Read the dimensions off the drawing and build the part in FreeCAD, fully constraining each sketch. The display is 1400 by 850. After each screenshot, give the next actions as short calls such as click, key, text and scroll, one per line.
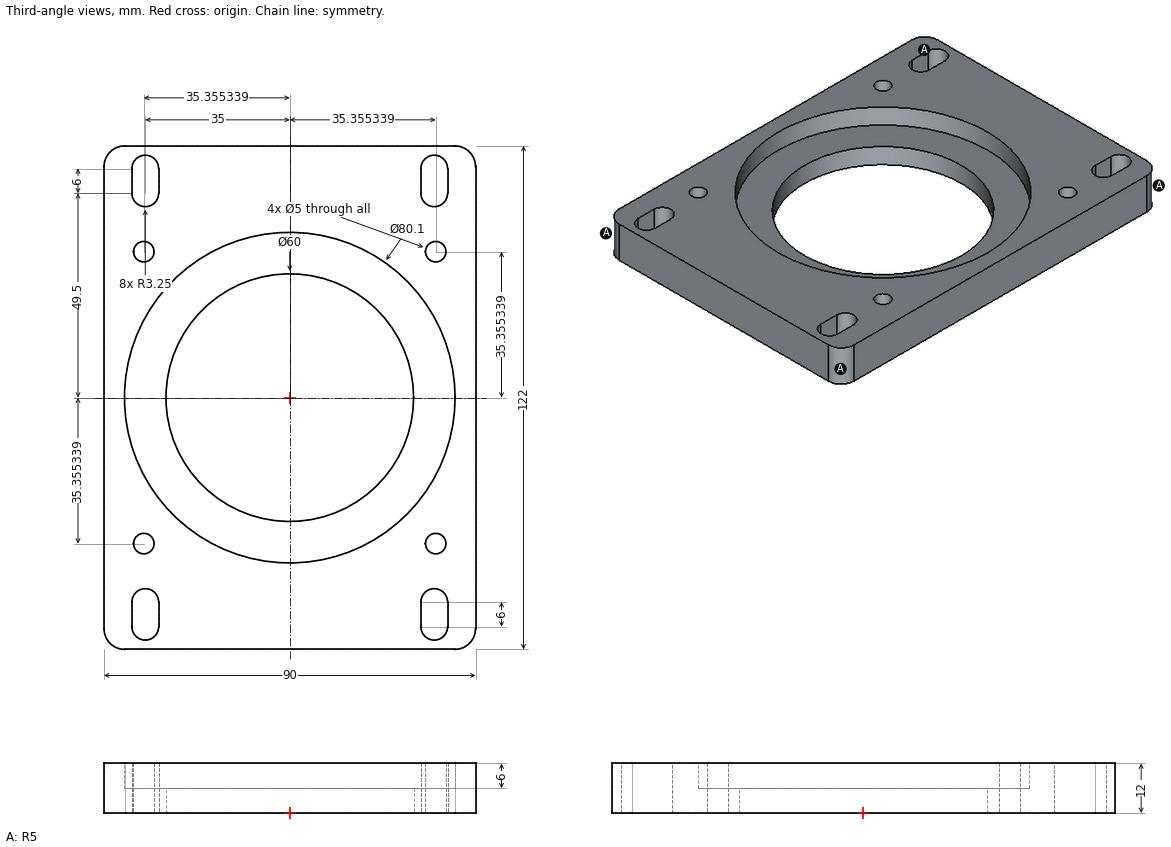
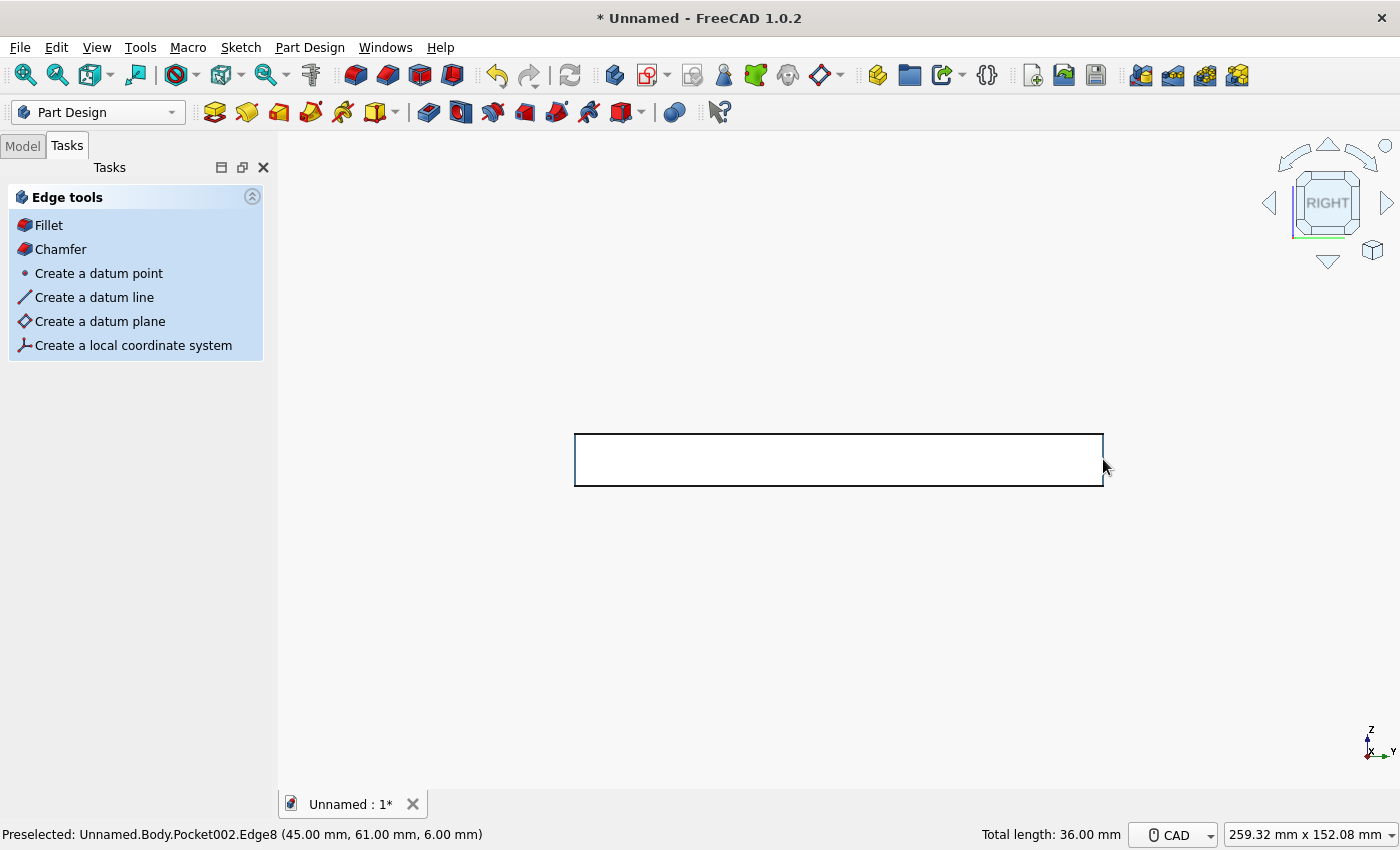
key(5)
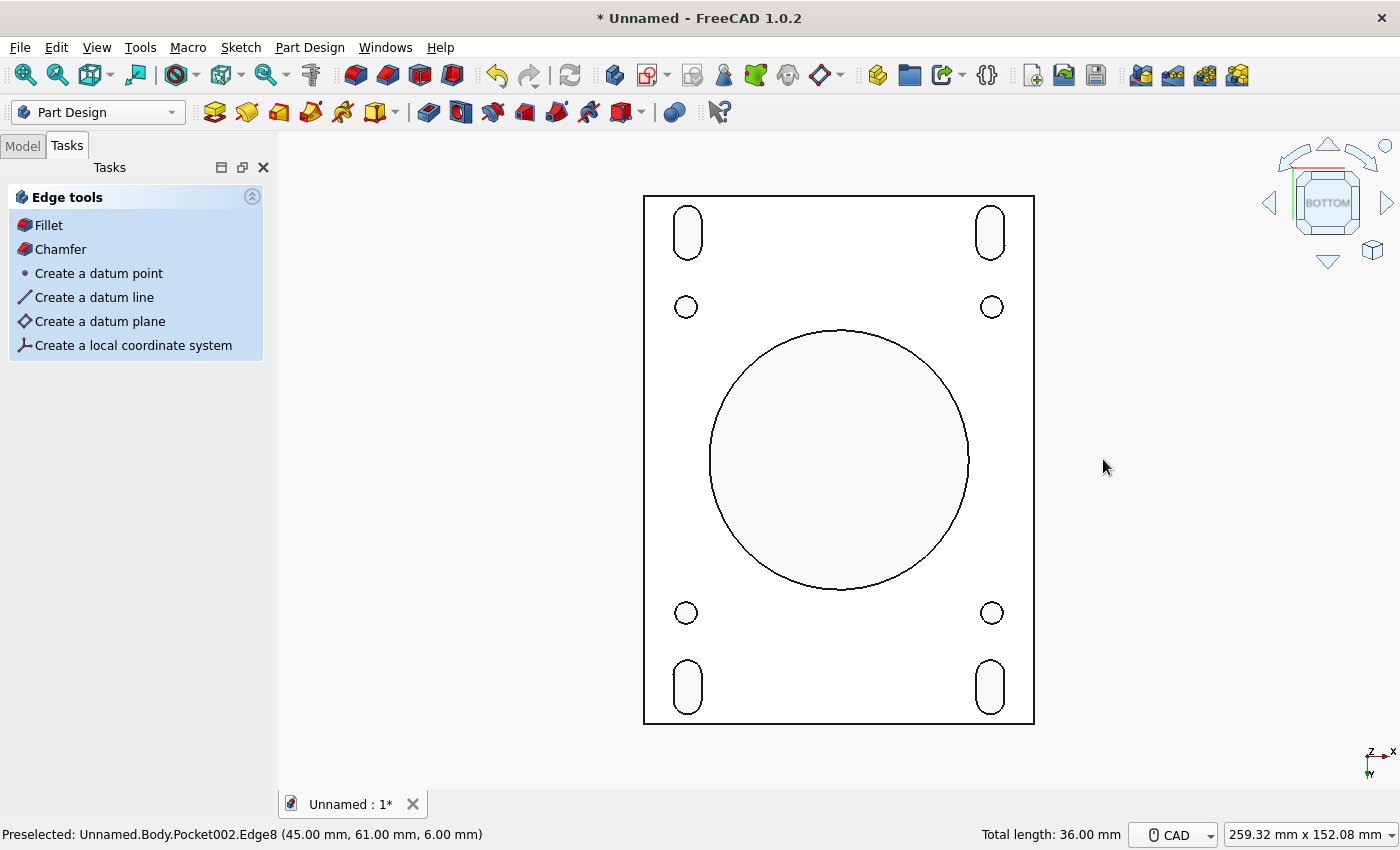
key(4)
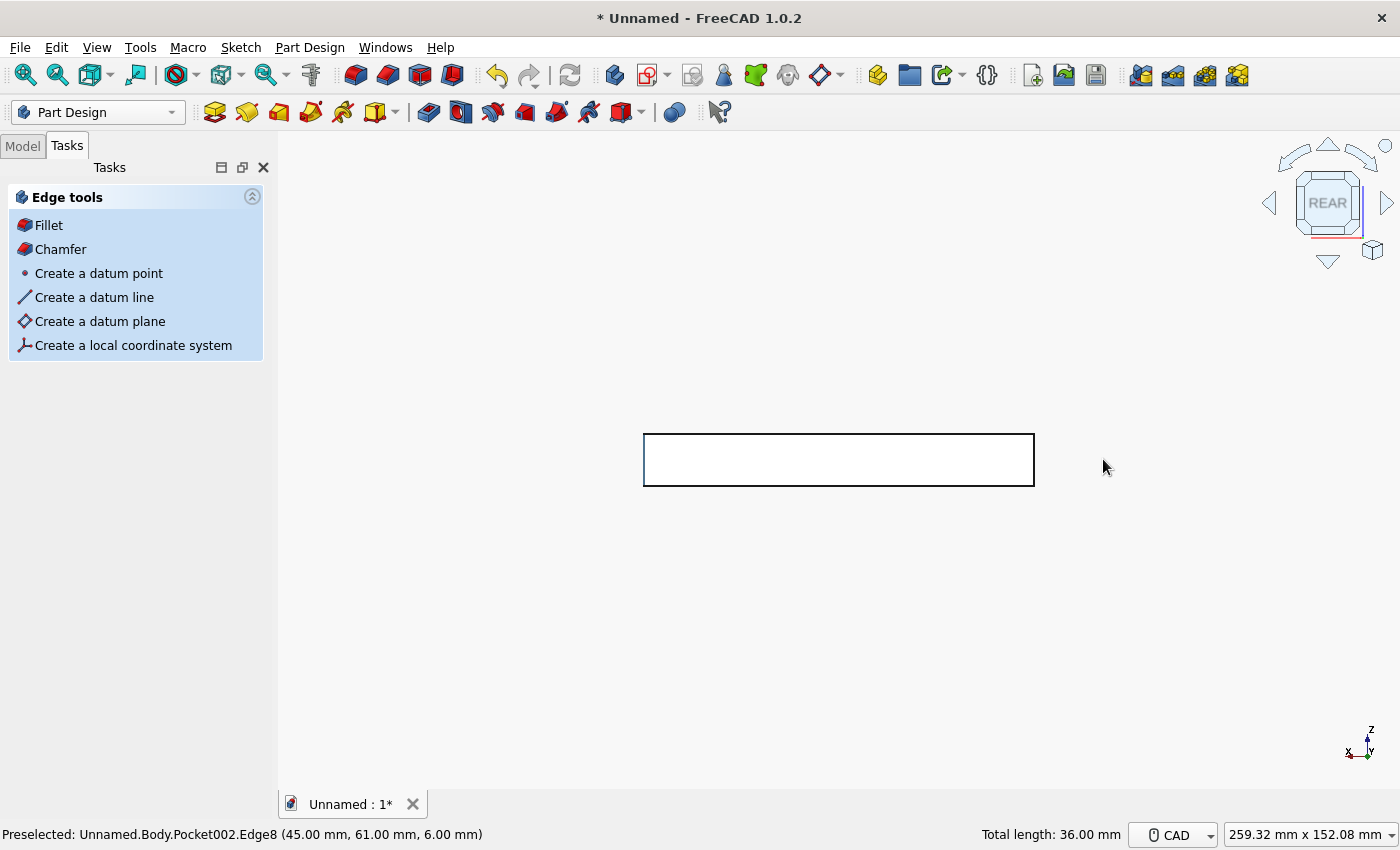
click(26, 76)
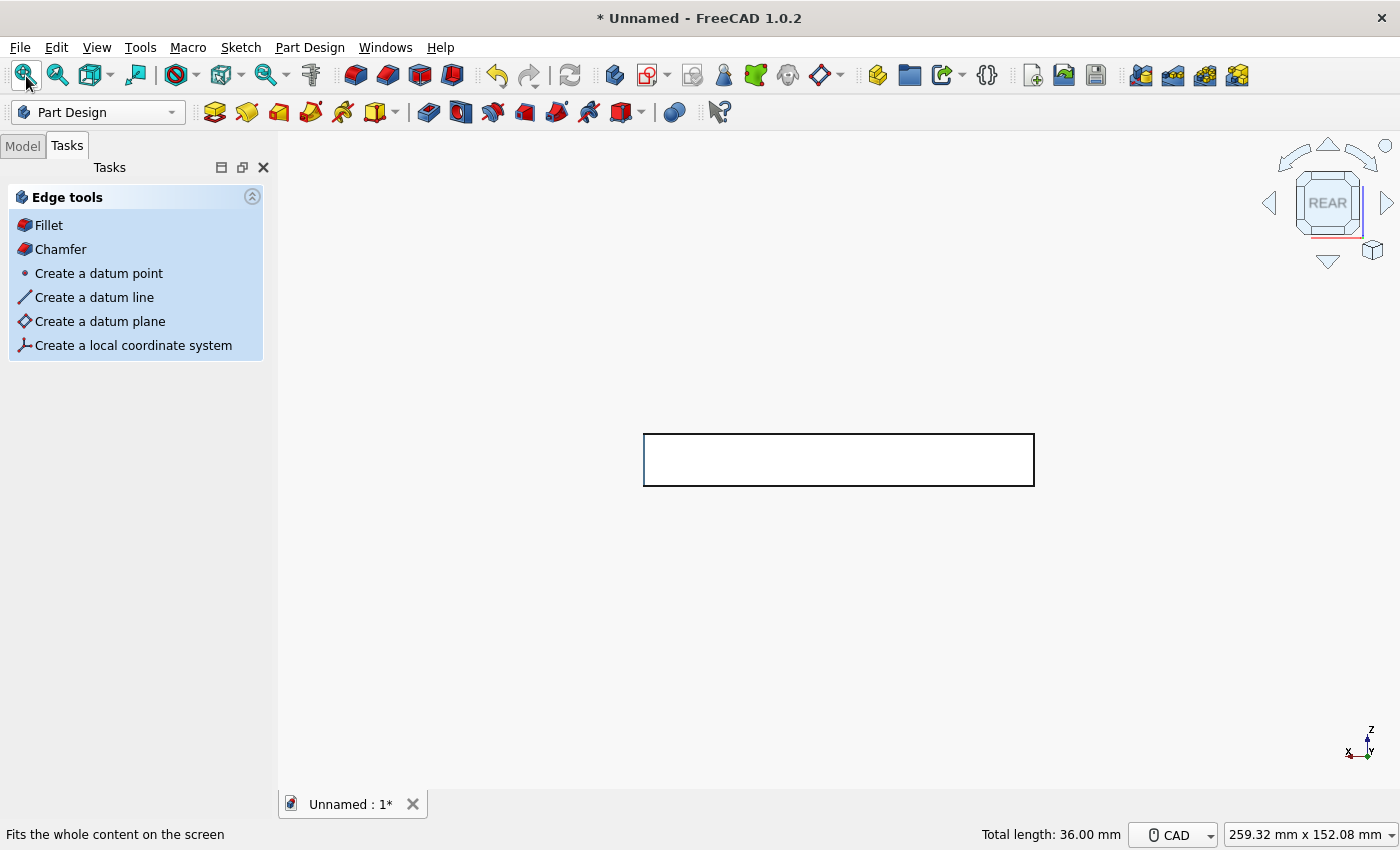
click(1034, 459, ctrl)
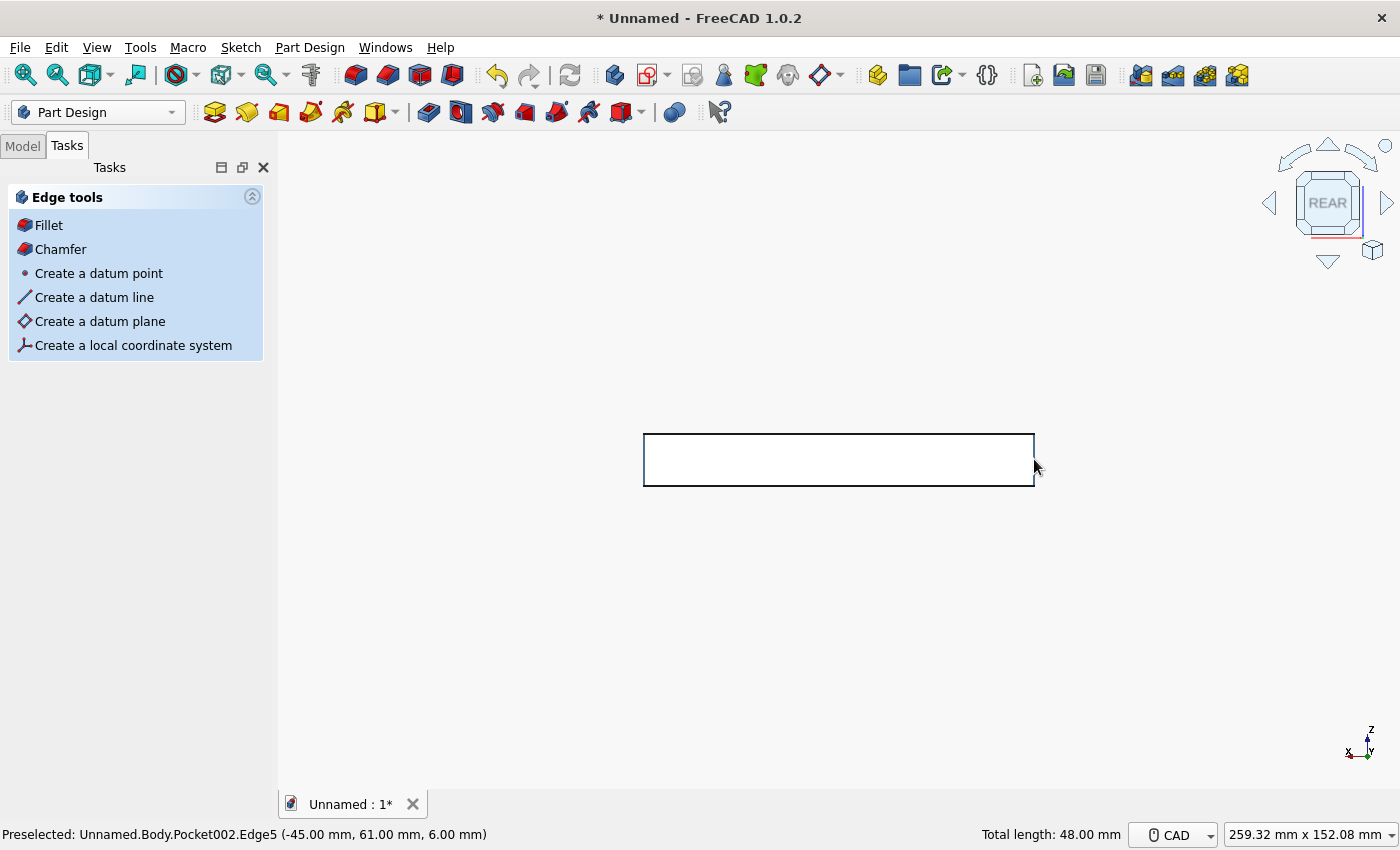
click(356, 76)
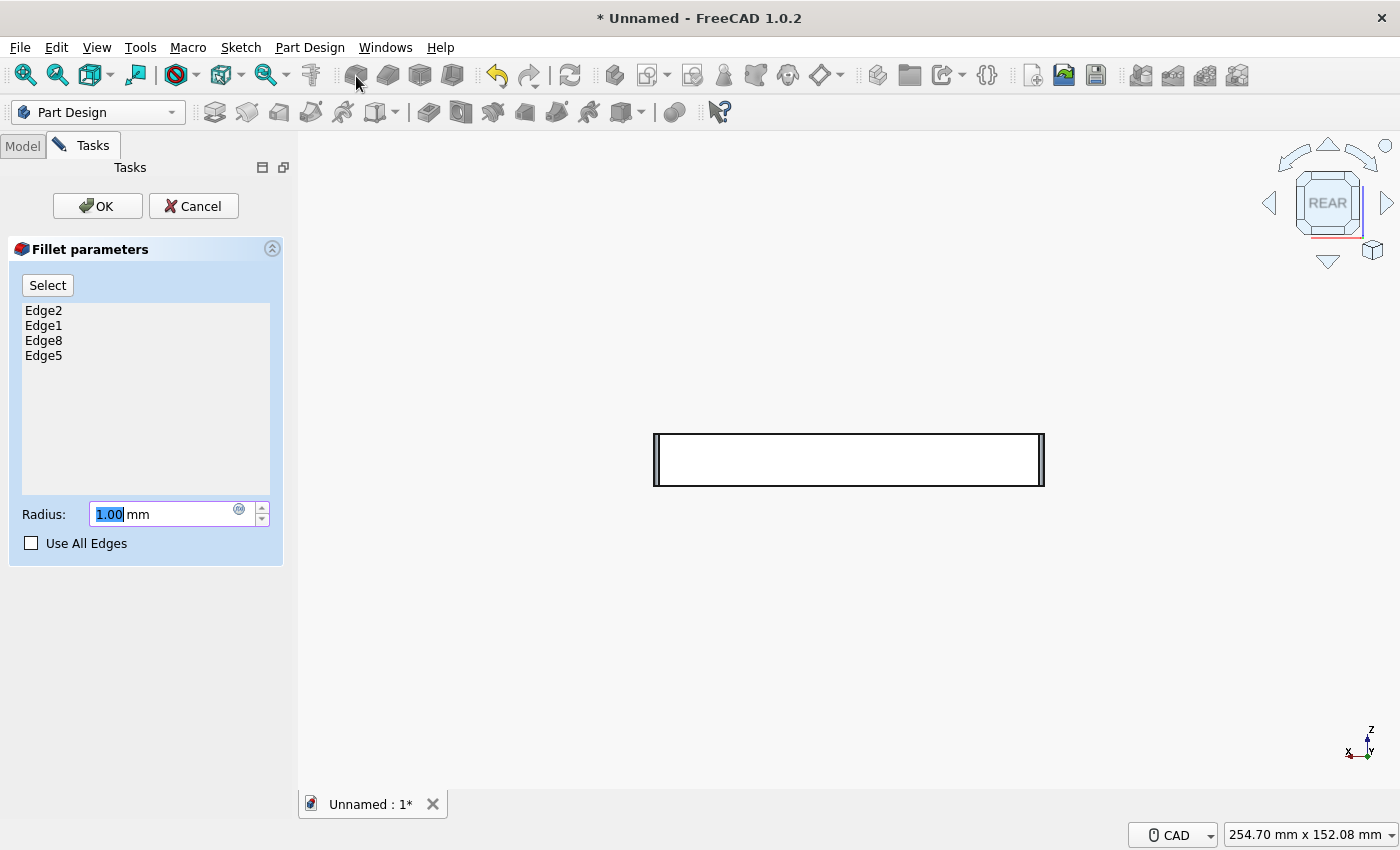
text(5)
key(Tab)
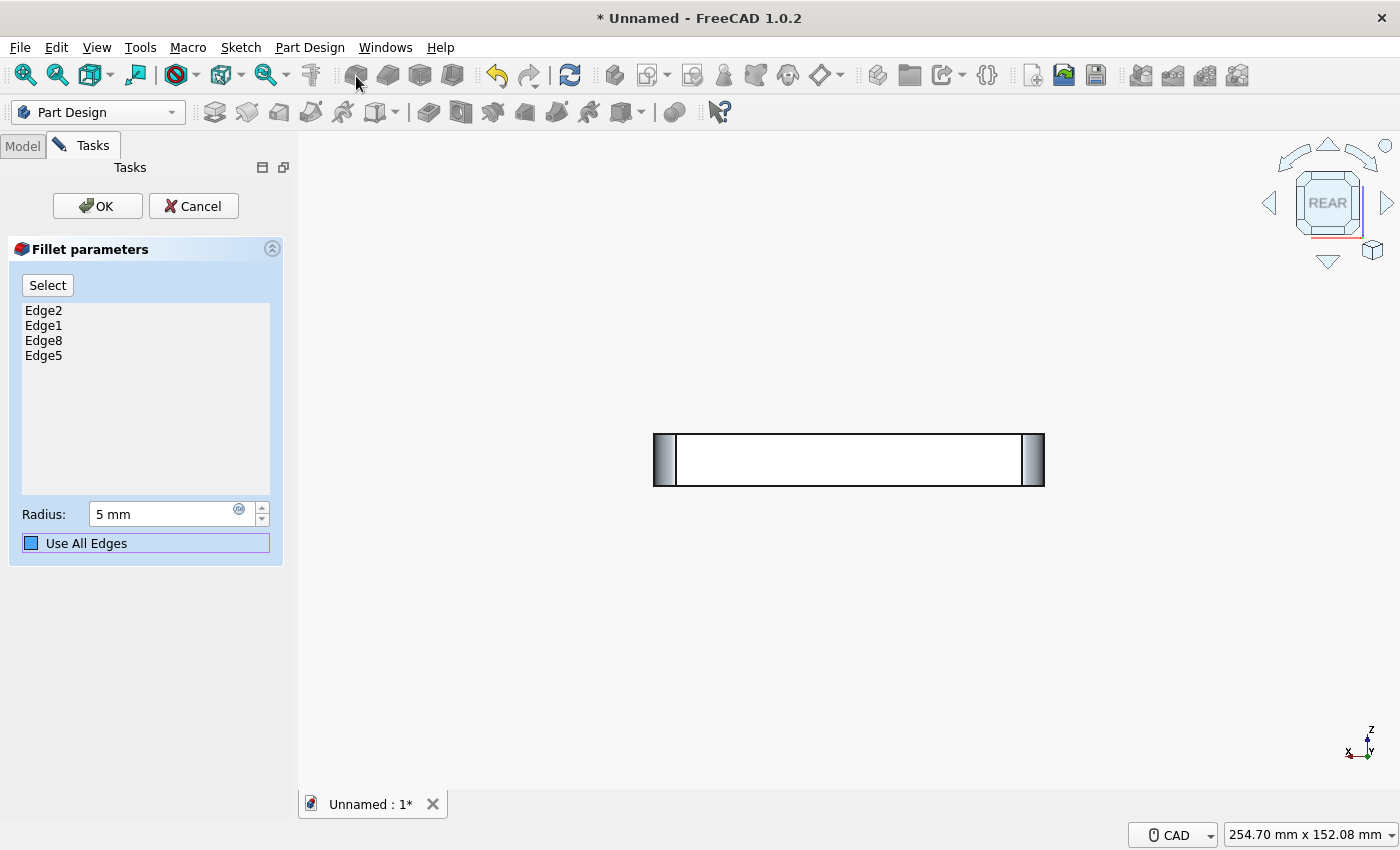
click(98, 206)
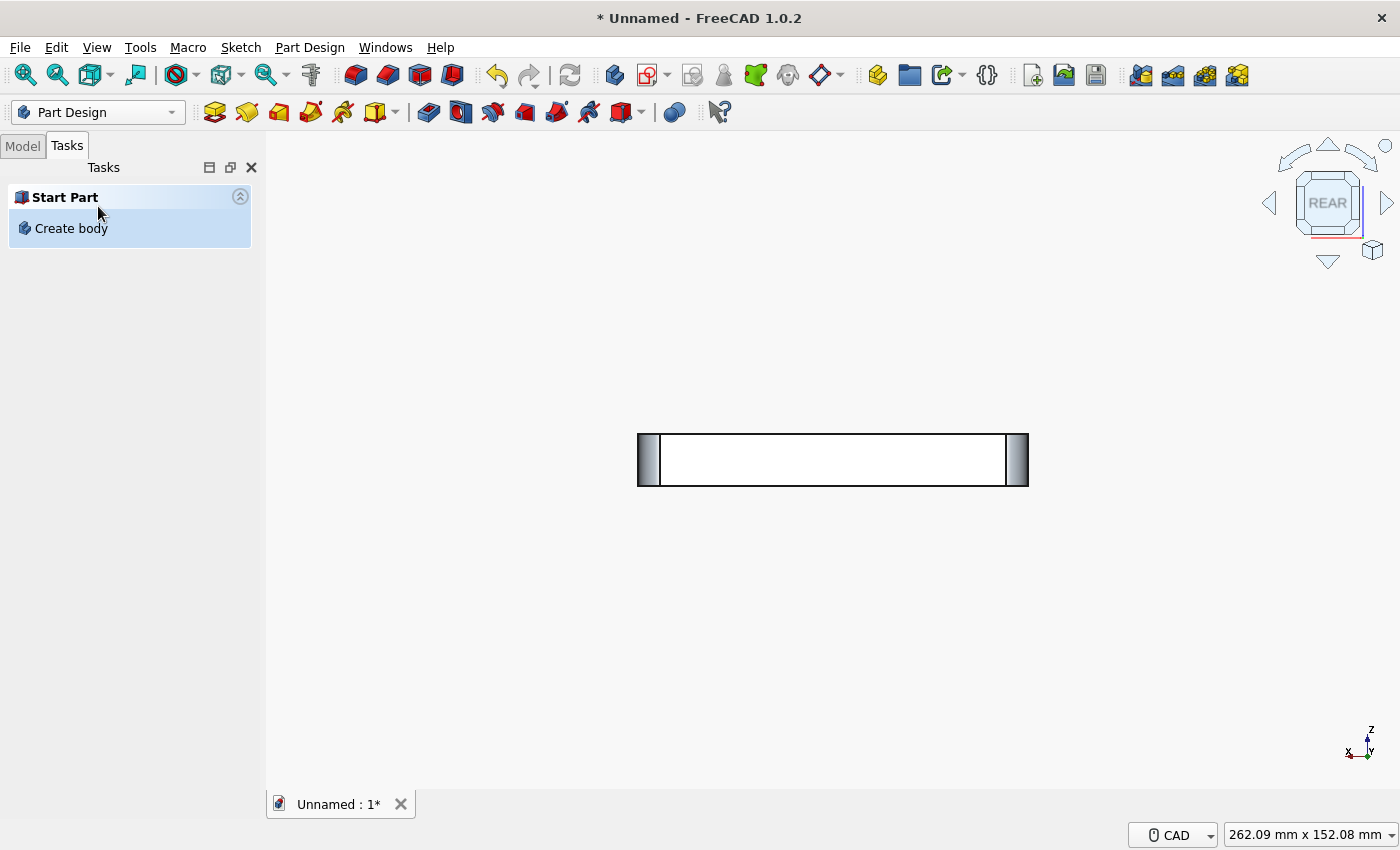
key(0)